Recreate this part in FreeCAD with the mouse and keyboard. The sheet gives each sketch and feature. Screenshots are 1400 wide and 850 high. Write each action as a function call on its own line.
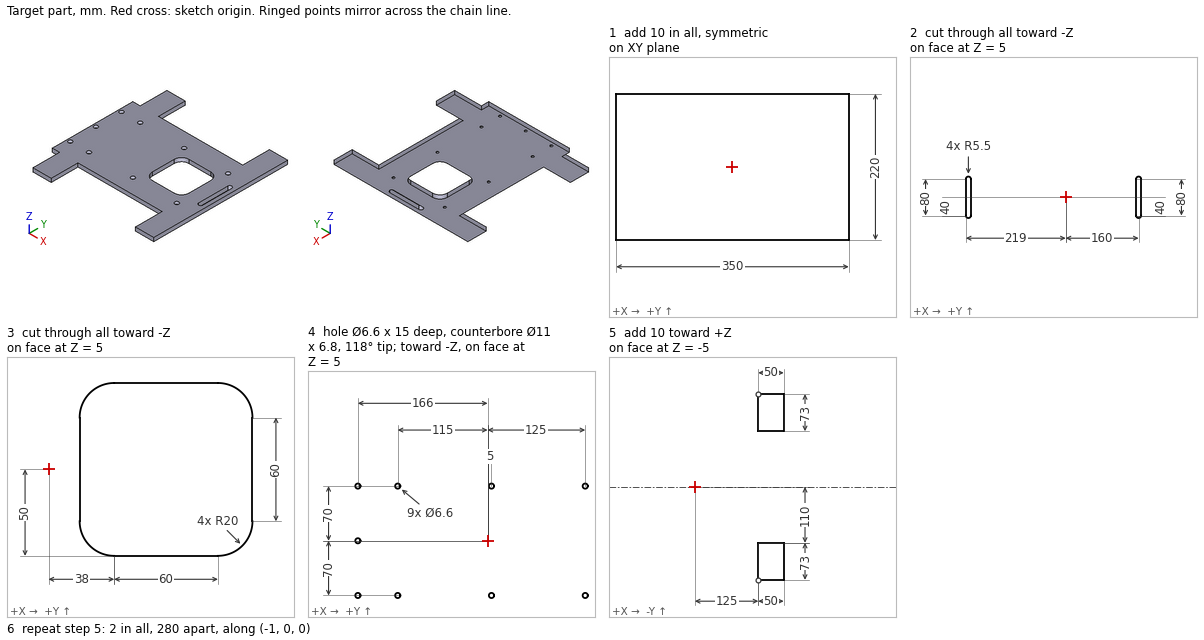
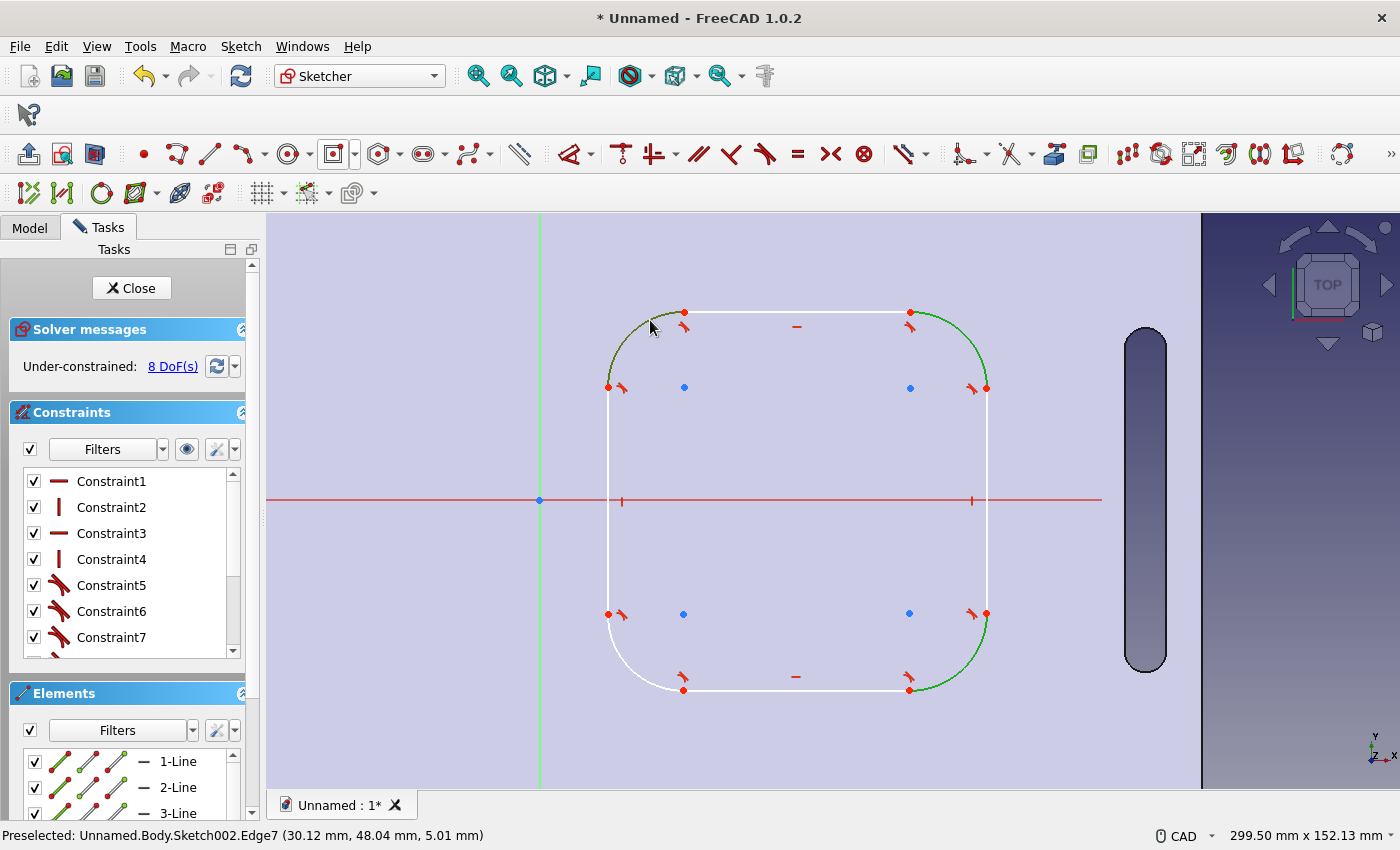
click(616, 649)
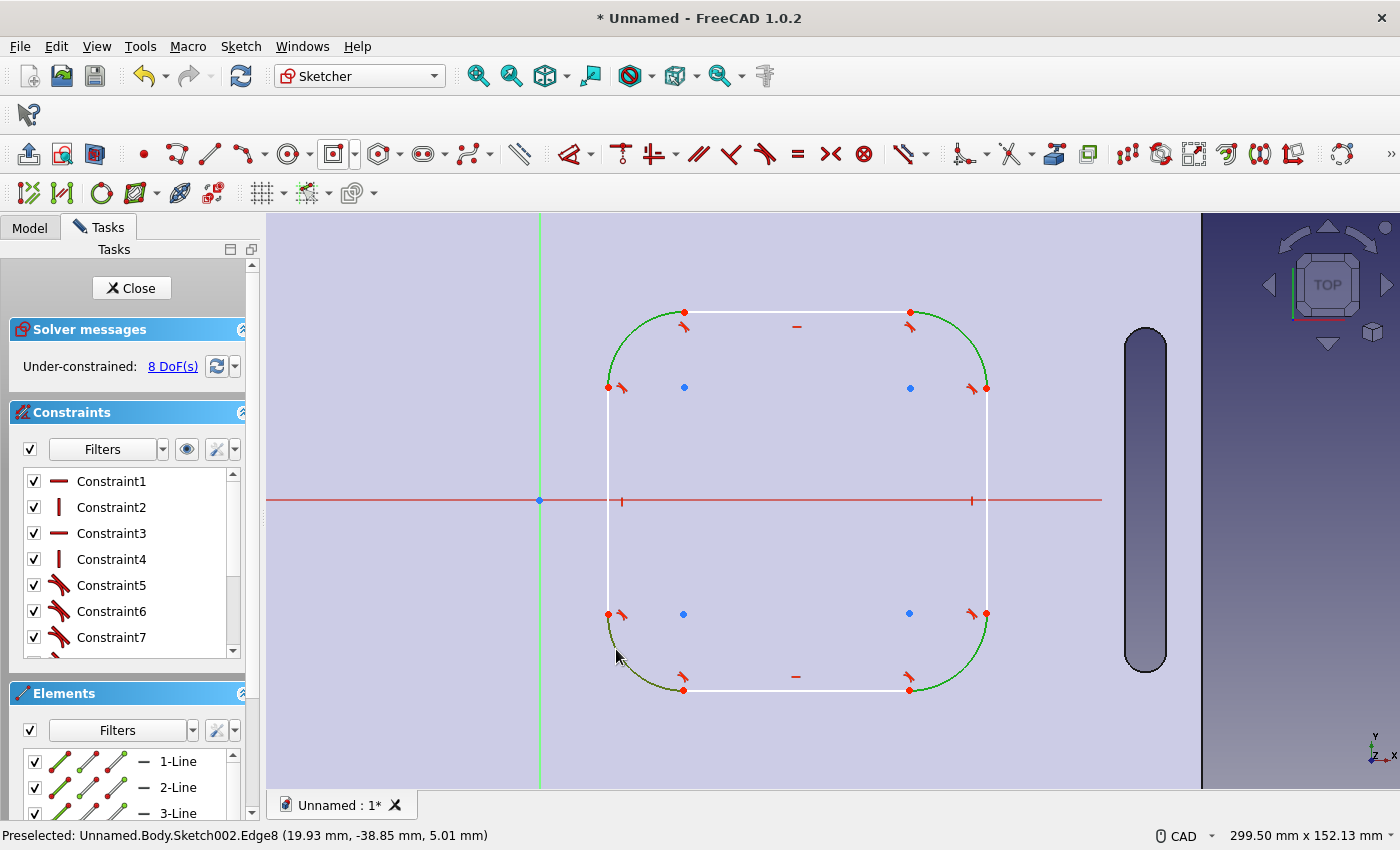
click(798, 154)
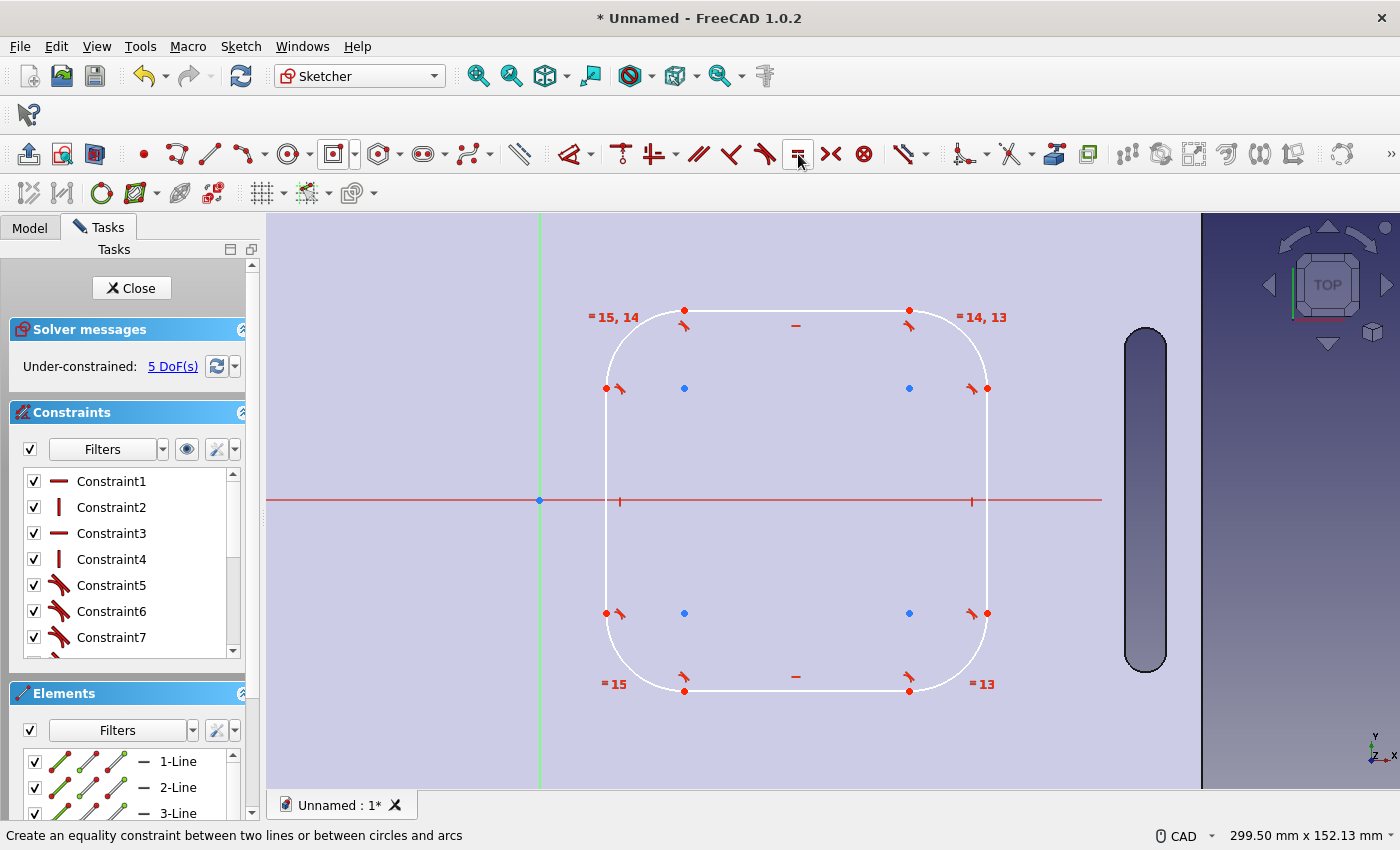
key(d)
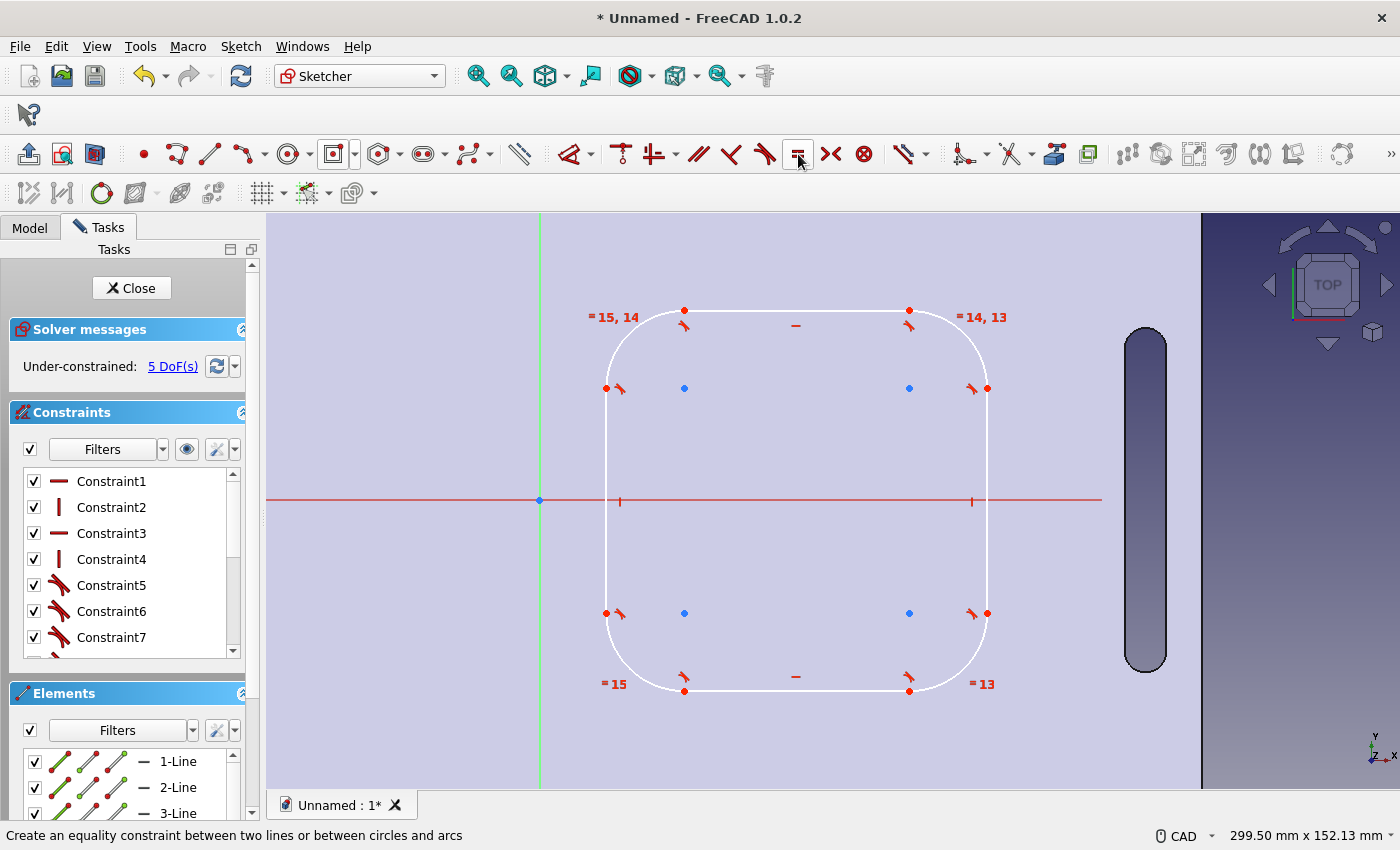
click(945, 683)
click(960, 711)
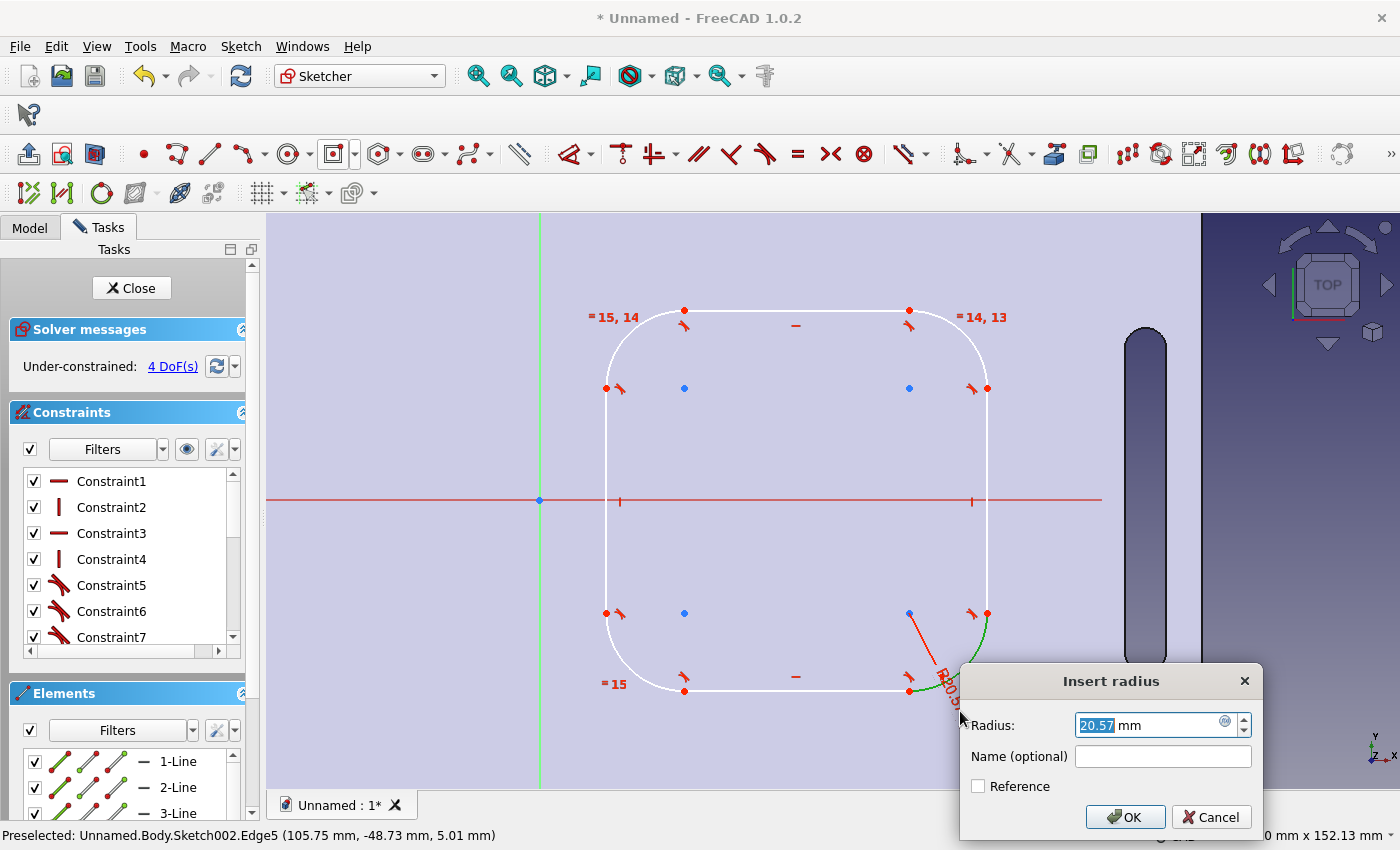
text(20)
key(Return)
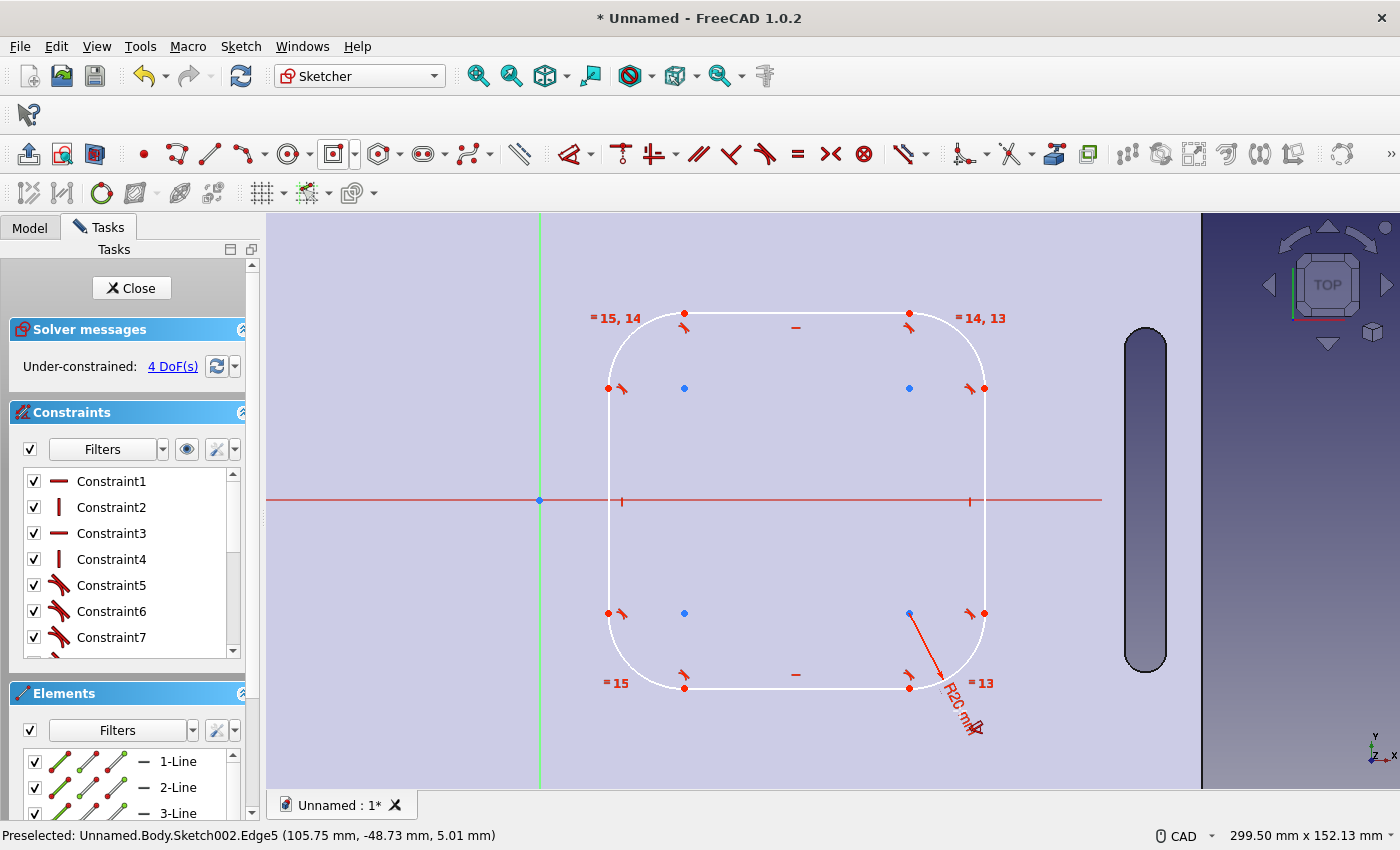
click(752, 689)
click(797, 723)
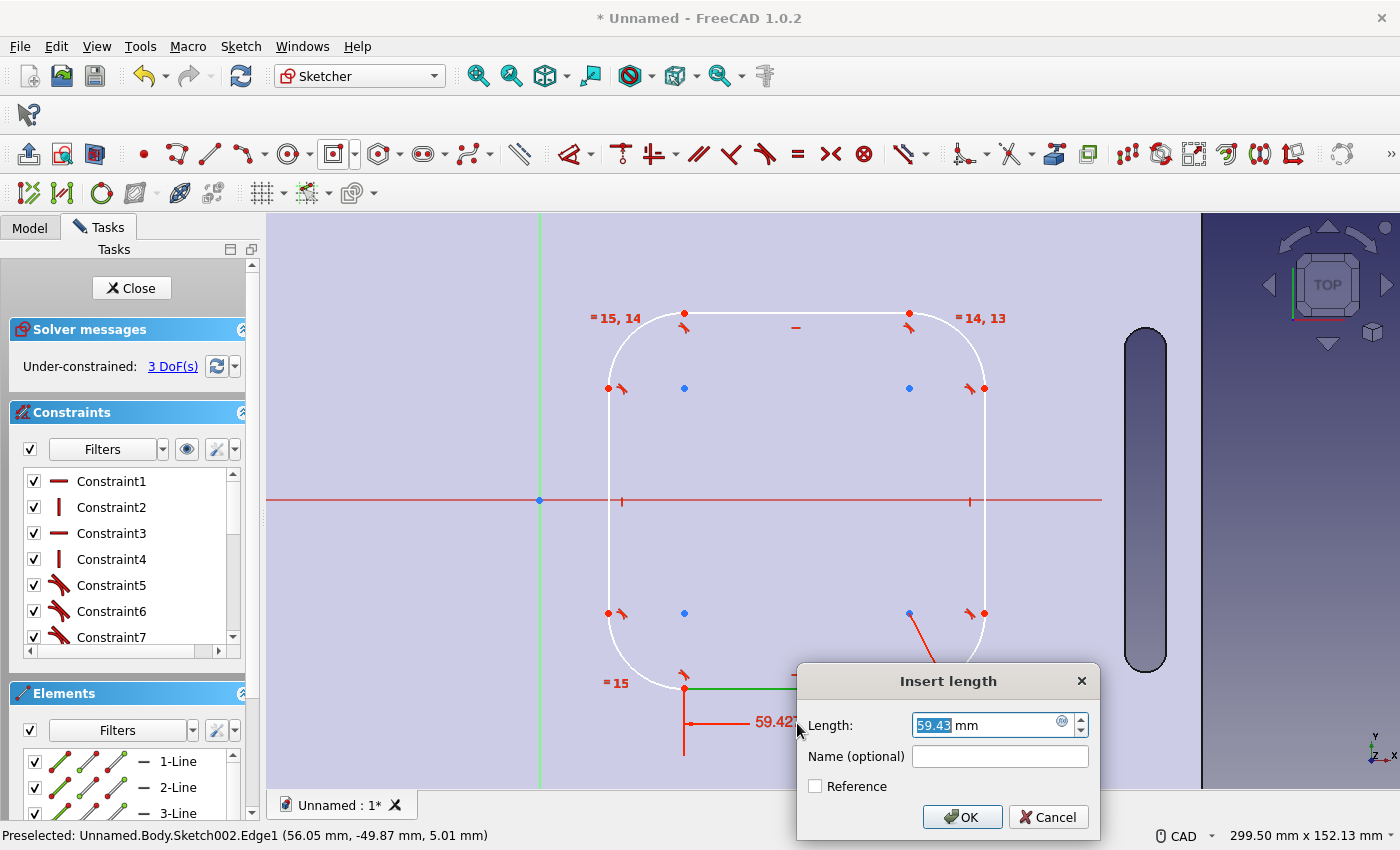
text(60)
key(Return)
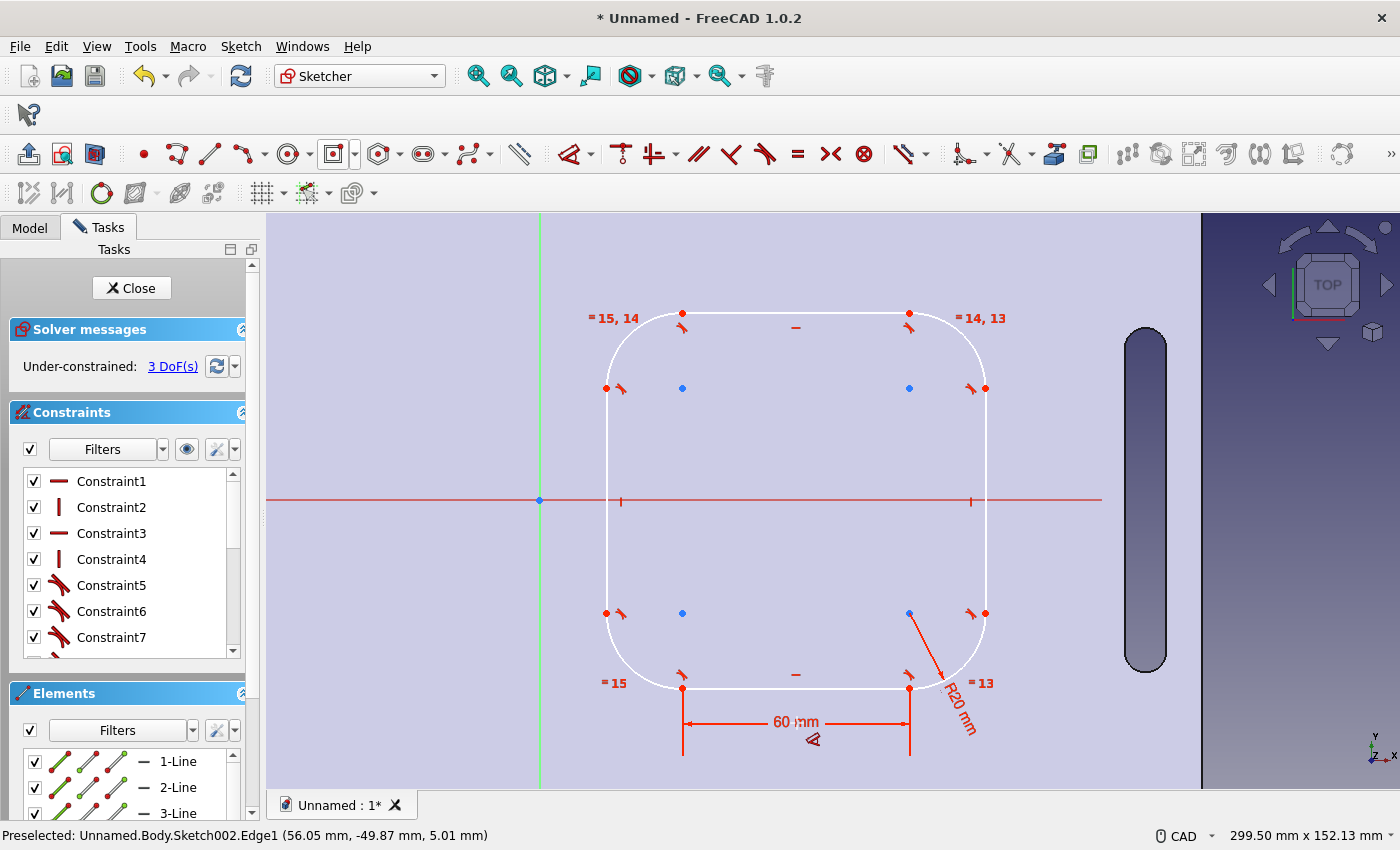
click(986, 546)
click(1020, 449)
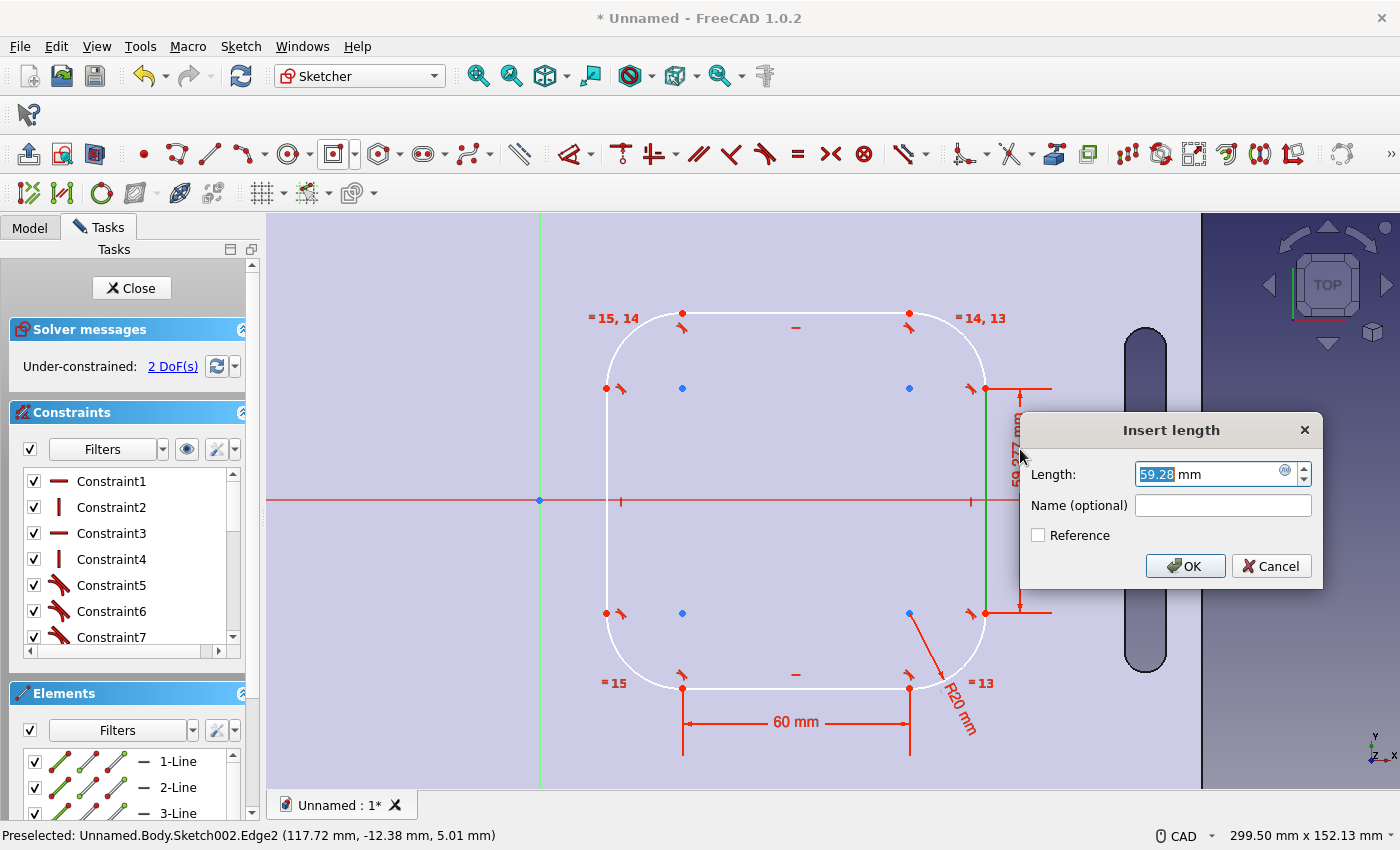
text(60)
key(Return)